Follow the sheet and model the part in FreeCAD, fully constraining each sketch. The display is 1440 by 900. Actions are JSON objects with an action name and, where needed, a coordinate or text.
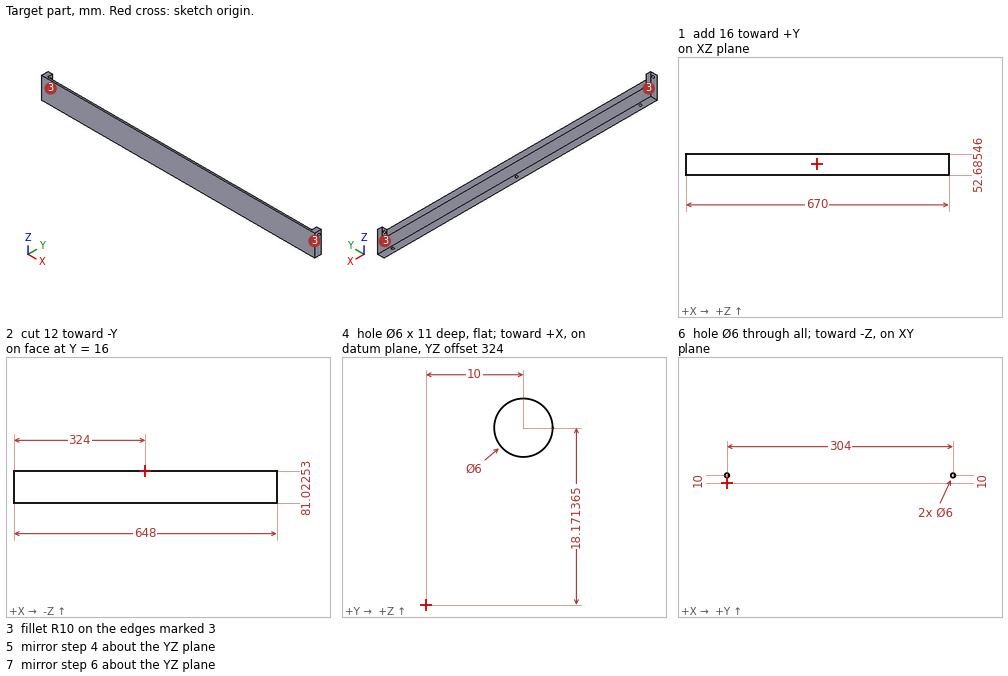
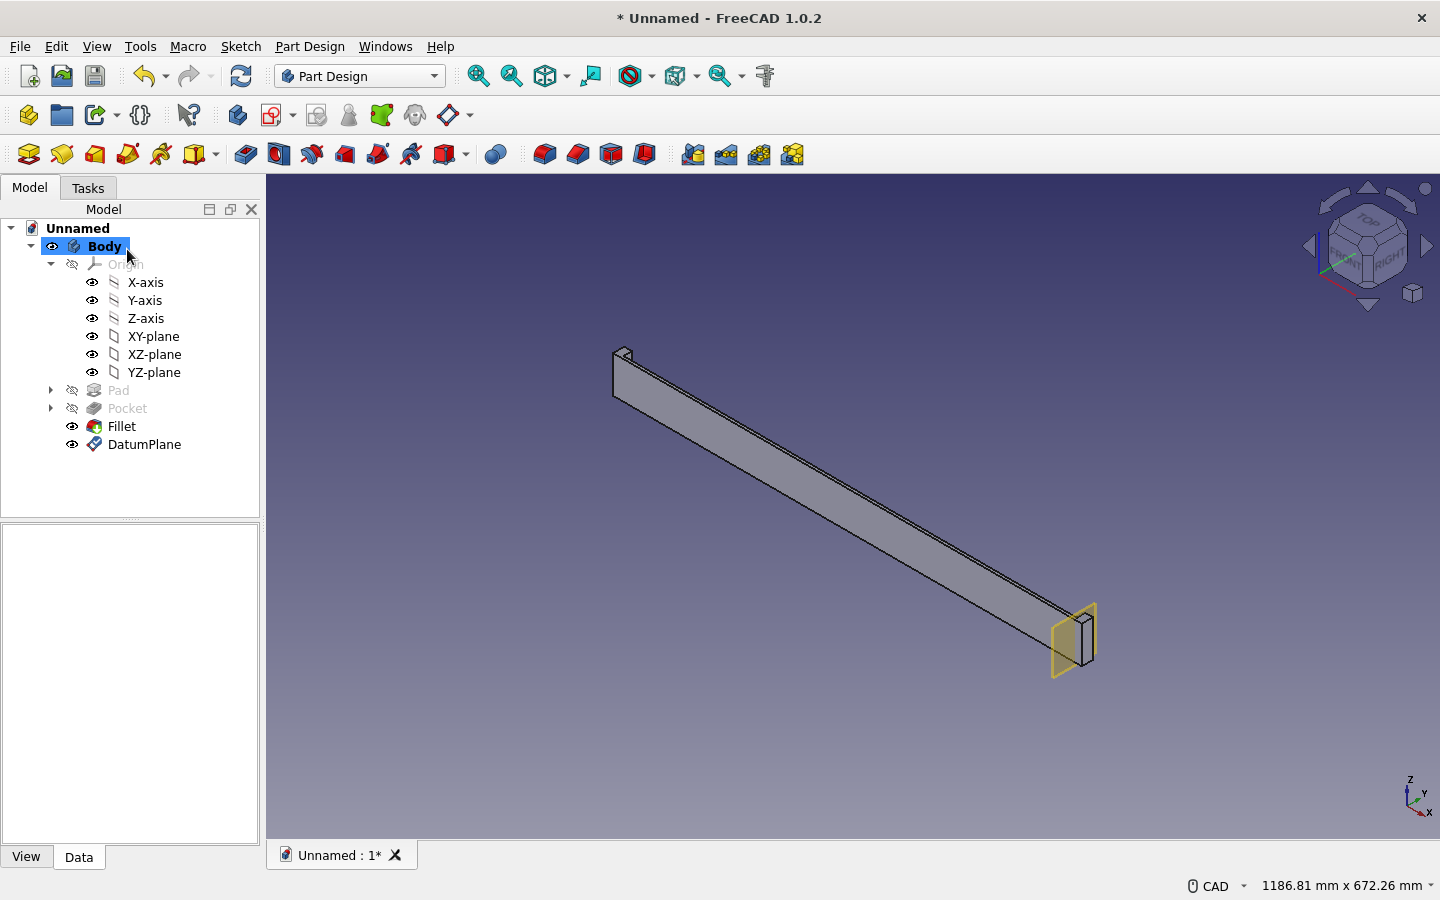
{"action": "left_click", "coordinate": [117, 444]}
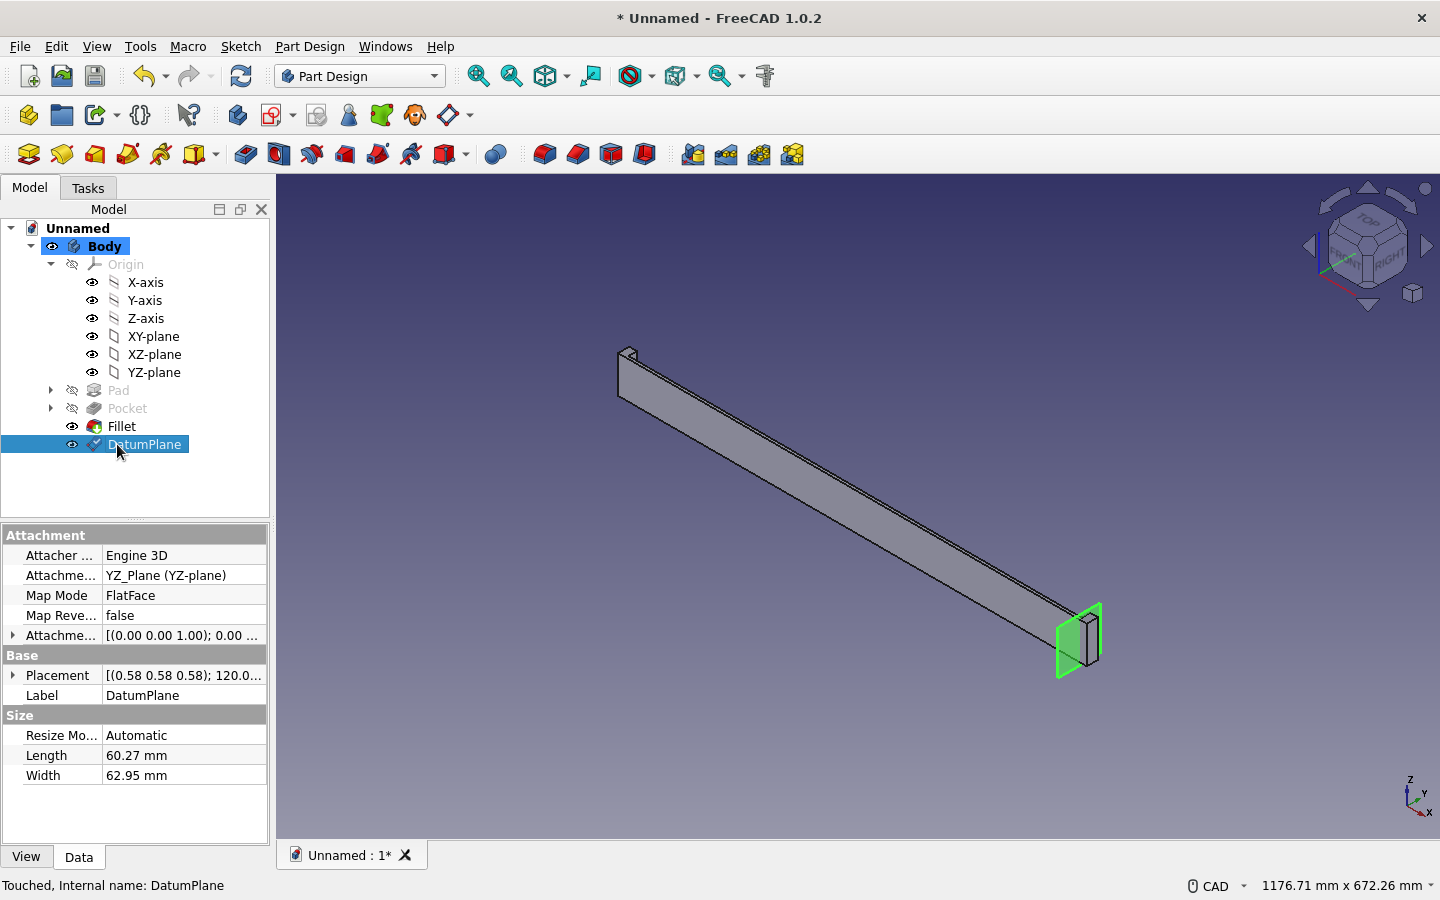
{"action": "left_click", "coordinate": [270, 116]}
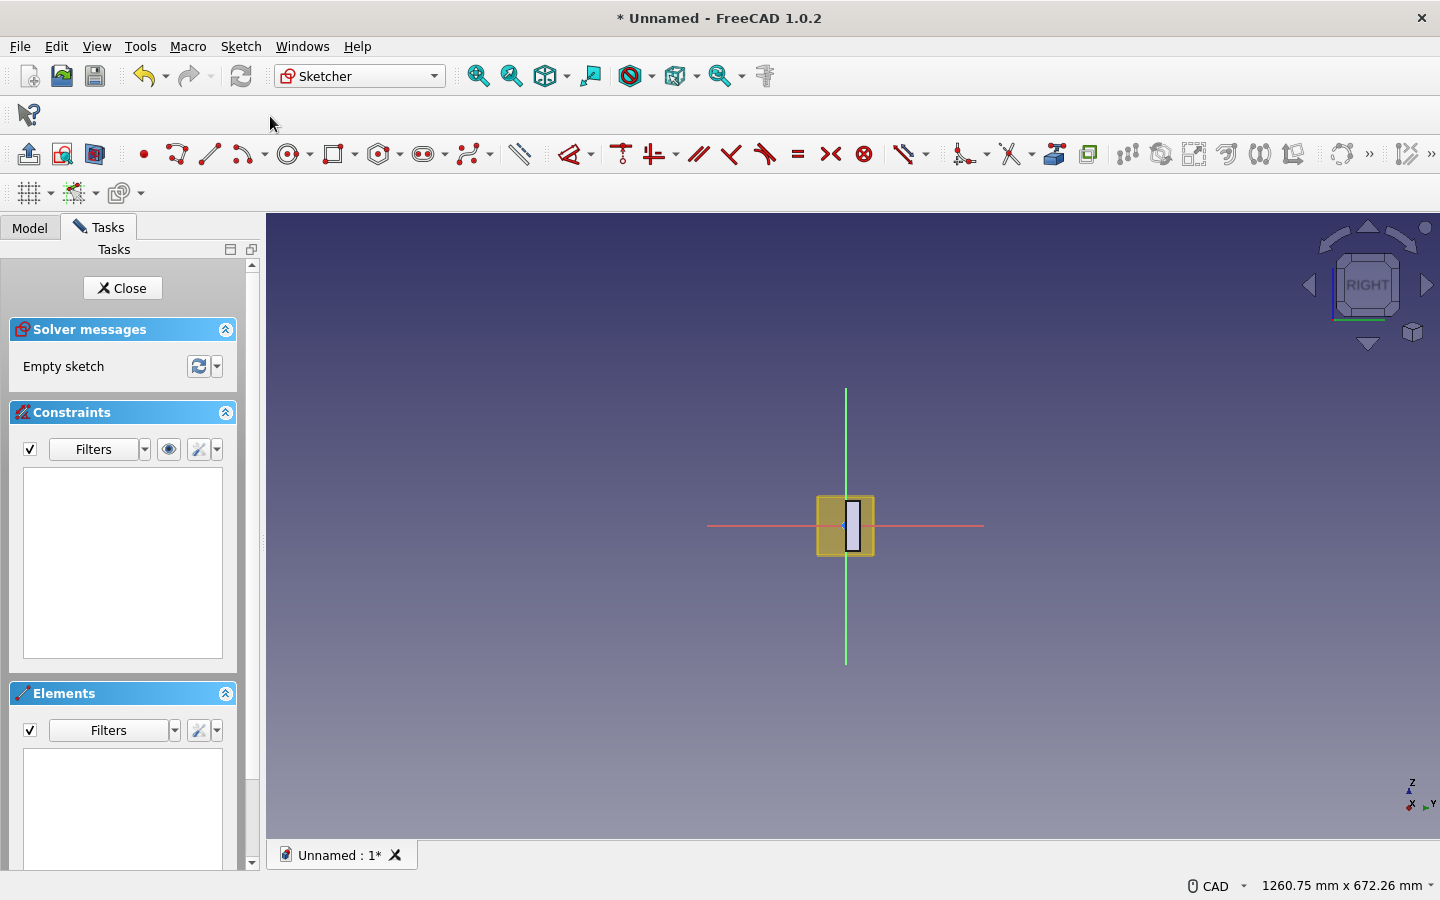
{"action": "left_click", "coordinate": [95, 154]}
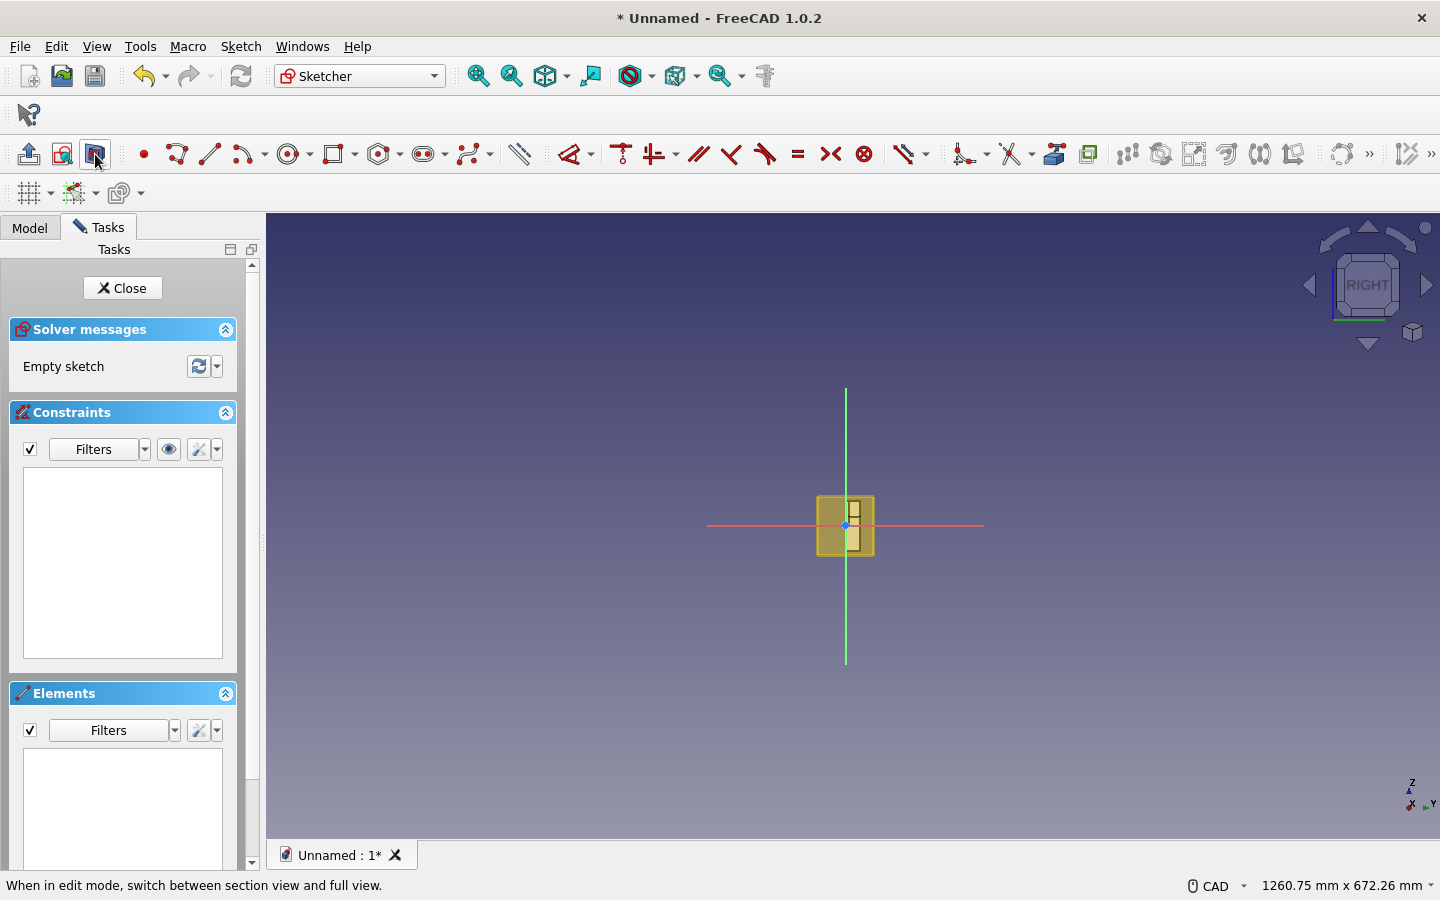
{"action": "scroll", "coordinate": [859, 508], "scroll_direction": "up", "scroll_amount": 15}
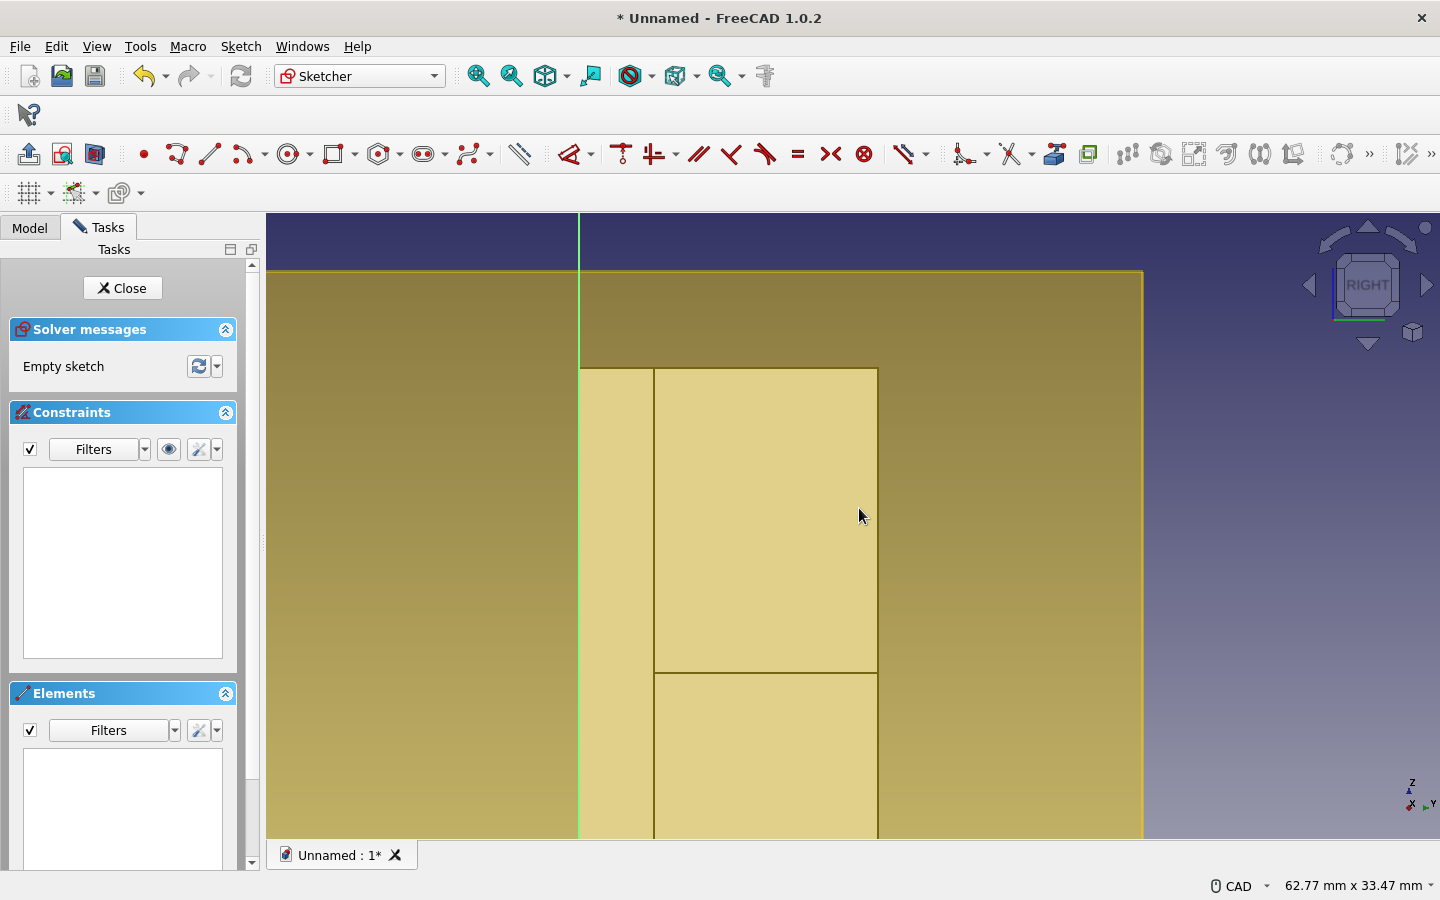
{"action": "scroll", "coordinate": [758, 518], "scroll_direction": "up", "scroll_amount": 6}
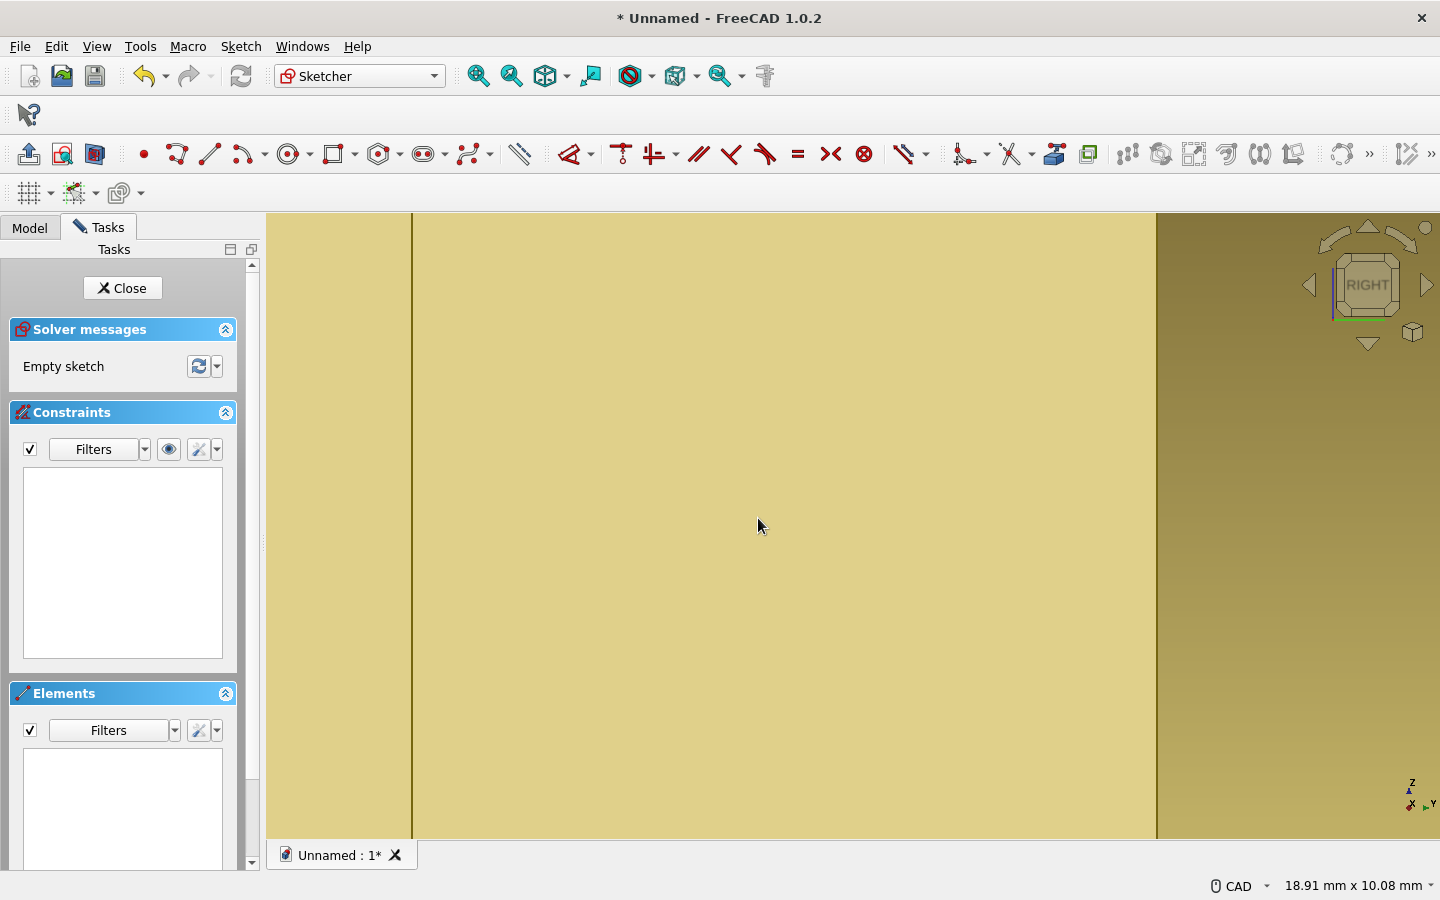
{"action": "key", "text": "g c"}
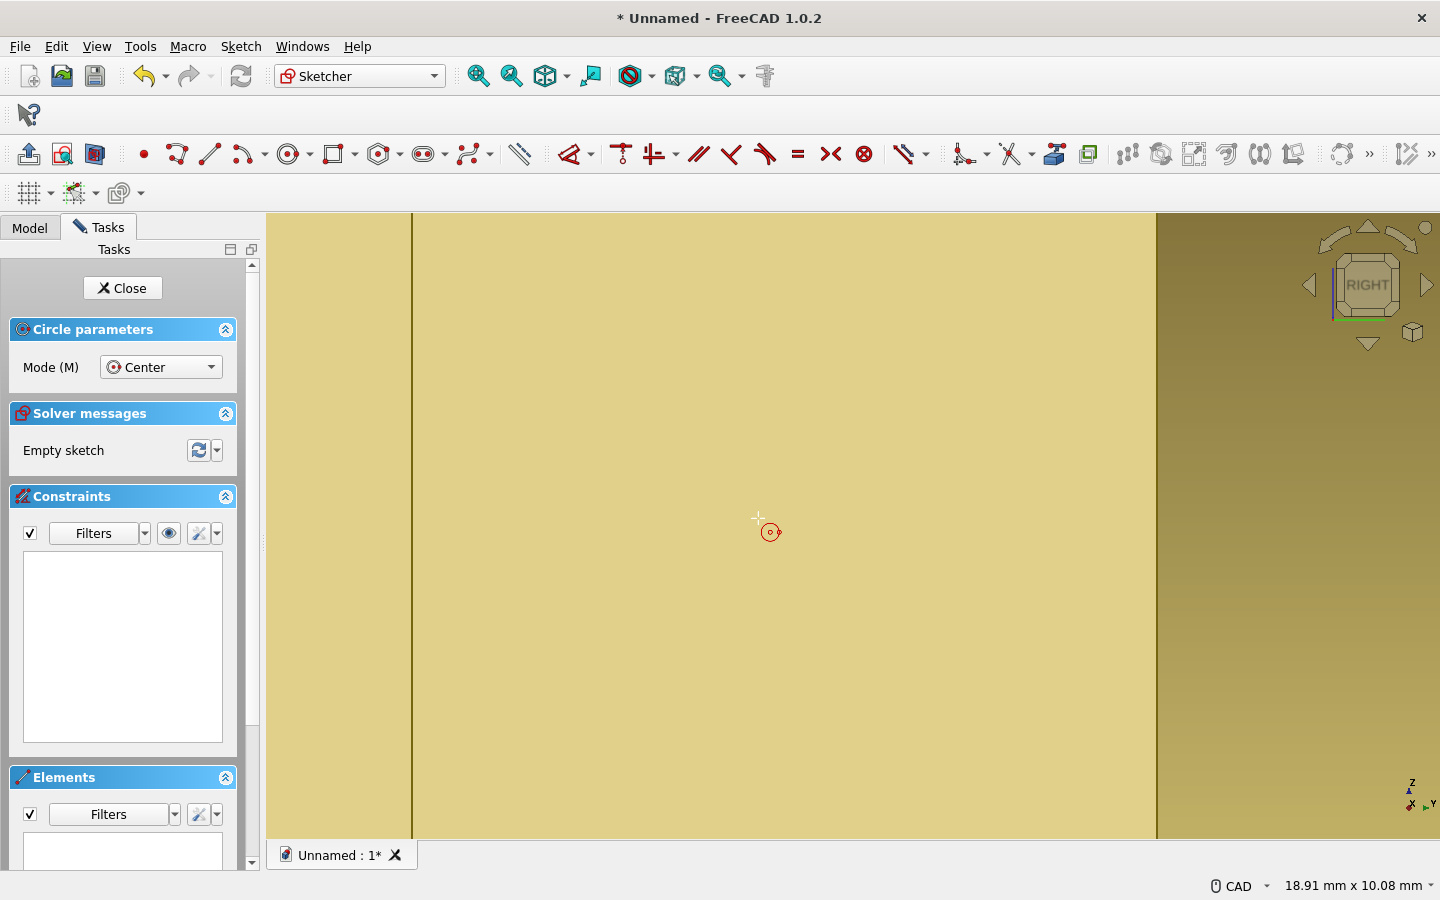
{"action": "left_click", "coordinate": [784, 526]}
{"action": "mouse_move", "coordinate": [916, 394]}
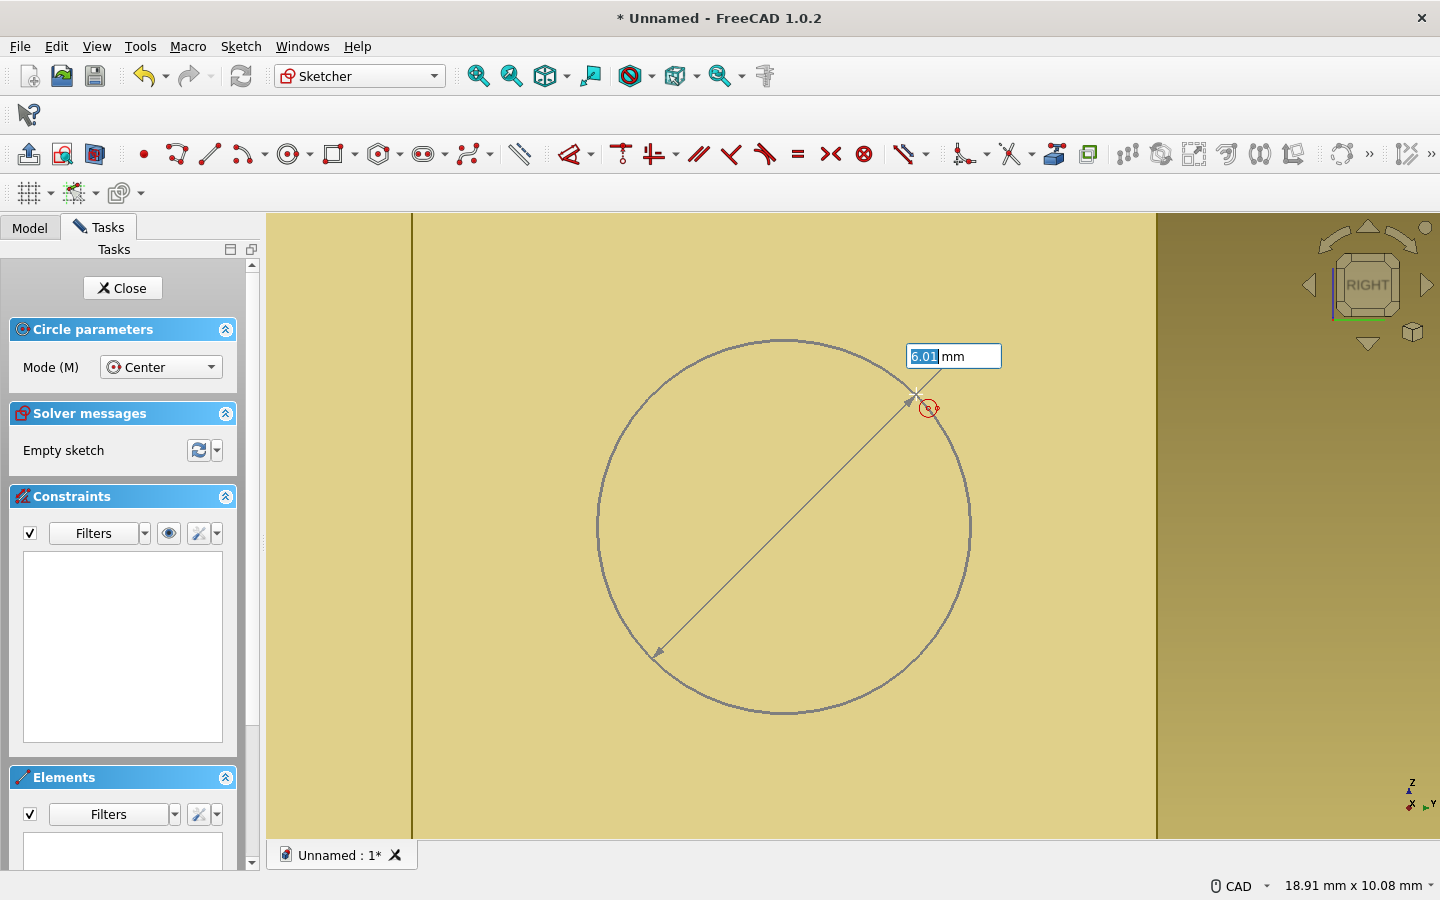
{"action": "type", "text": "6"}
{"action": "key", "text": "Return"}
{"action": "key", "text": "Escape"}